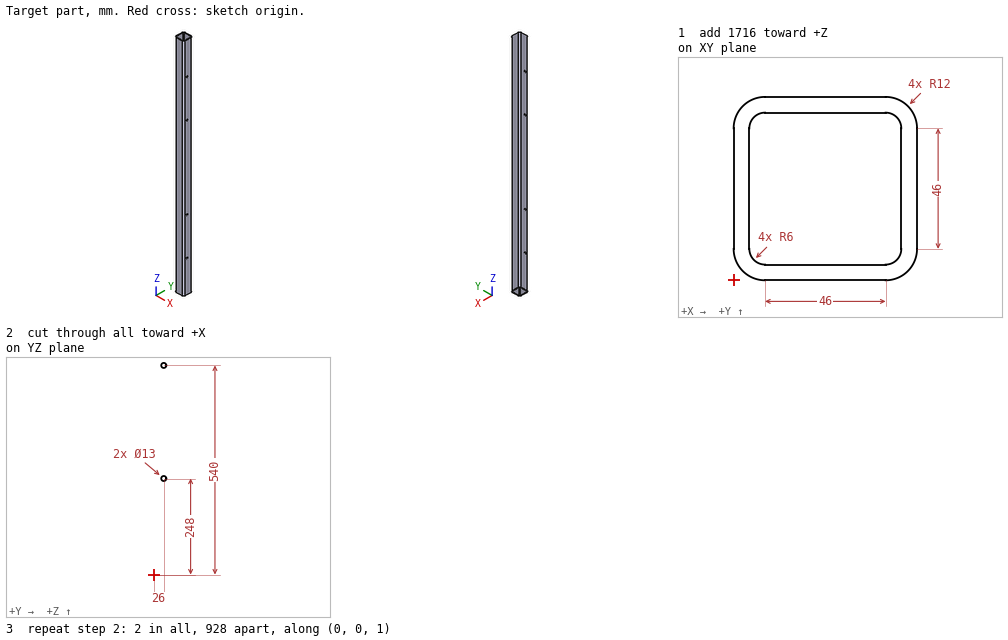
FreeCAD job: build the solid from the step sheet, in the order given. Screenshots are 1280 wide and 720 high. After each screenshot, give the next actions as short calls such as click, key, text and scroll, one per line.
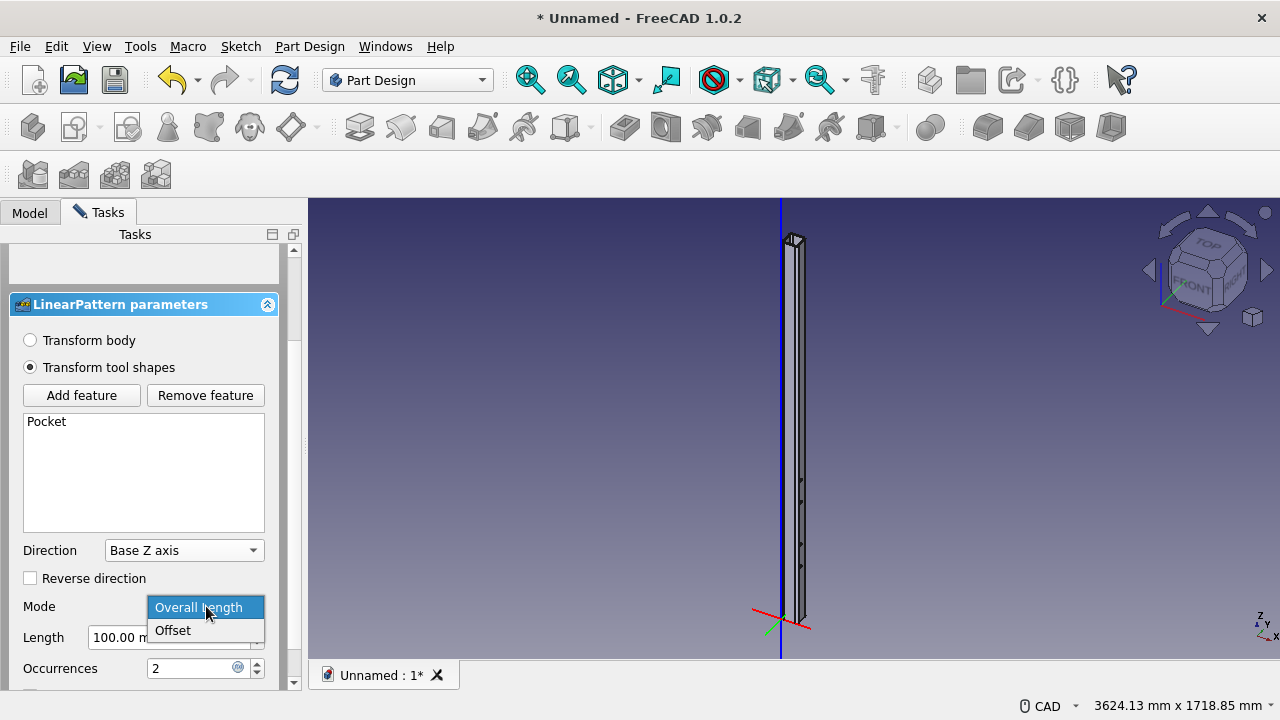
click(204, 630)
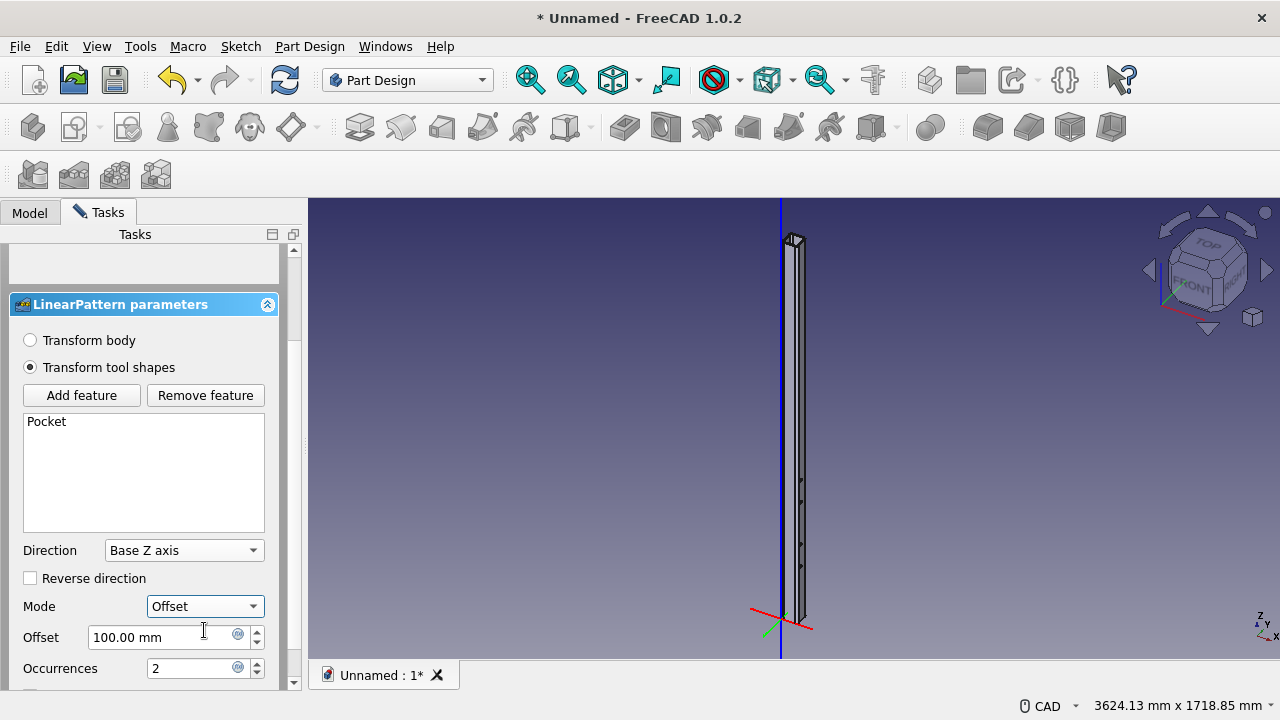
triple_click(170, 638)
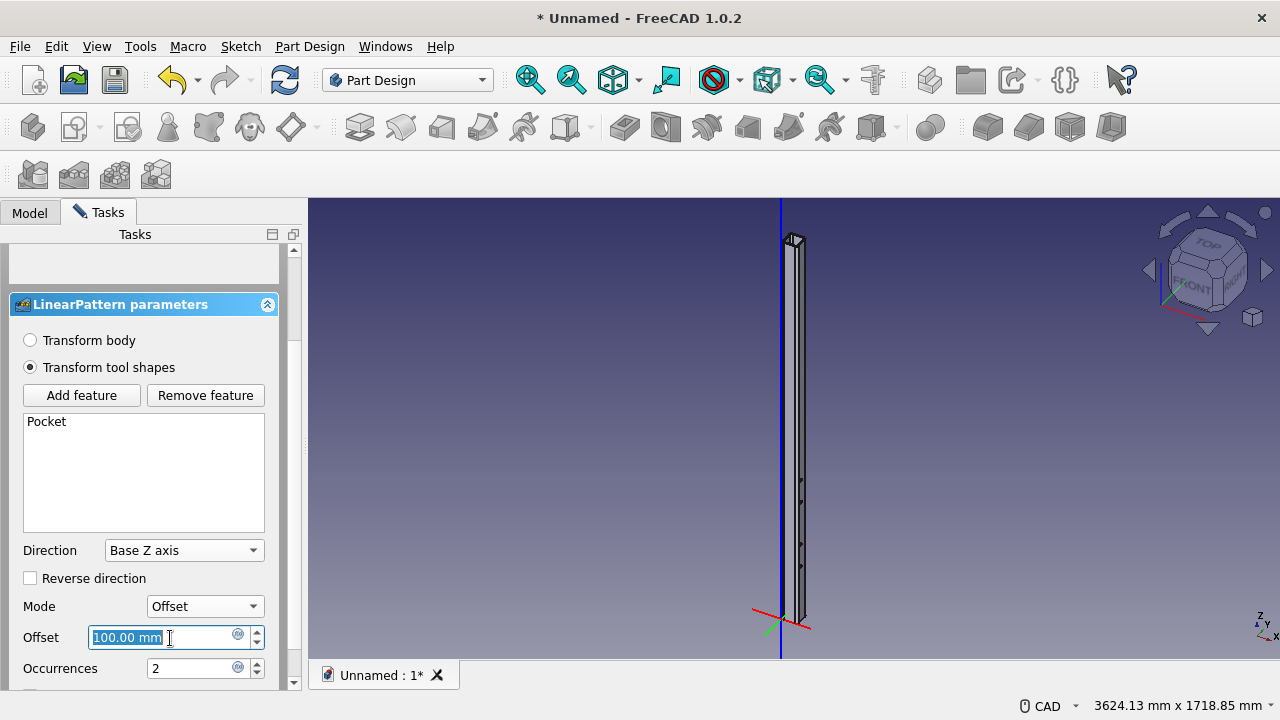
text(928)
key(Tab)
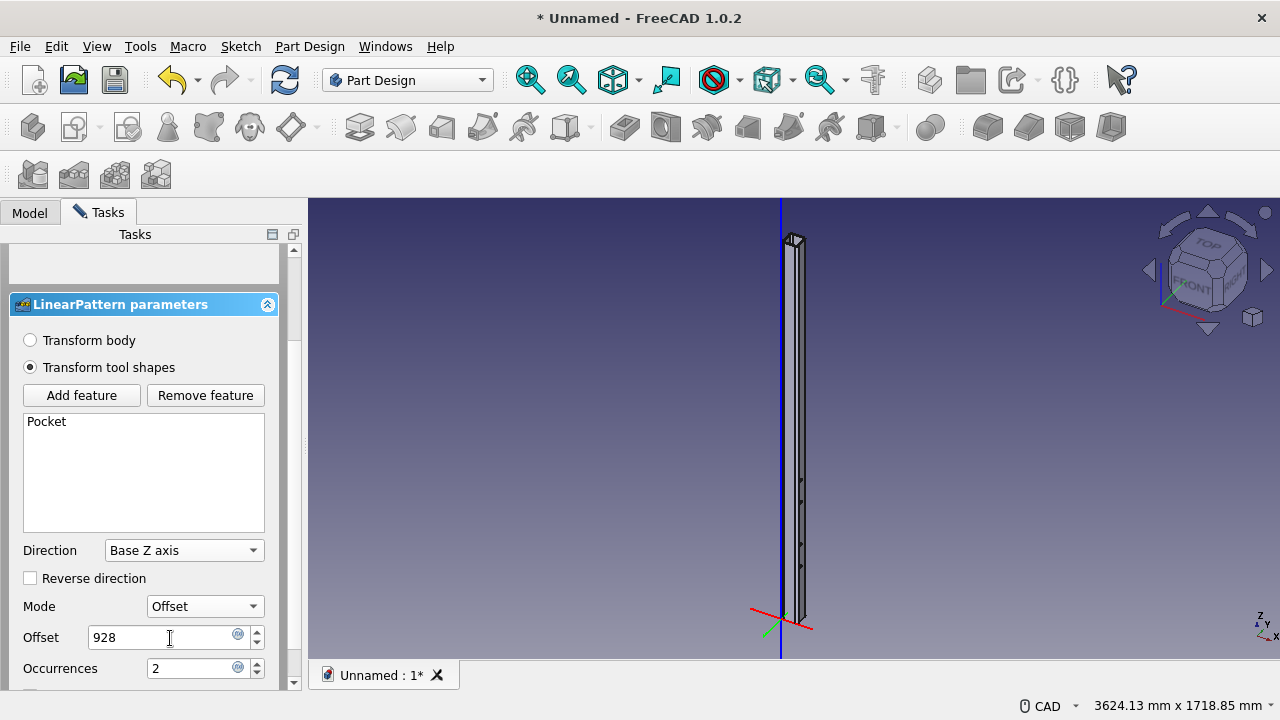
triple_click(199, 668)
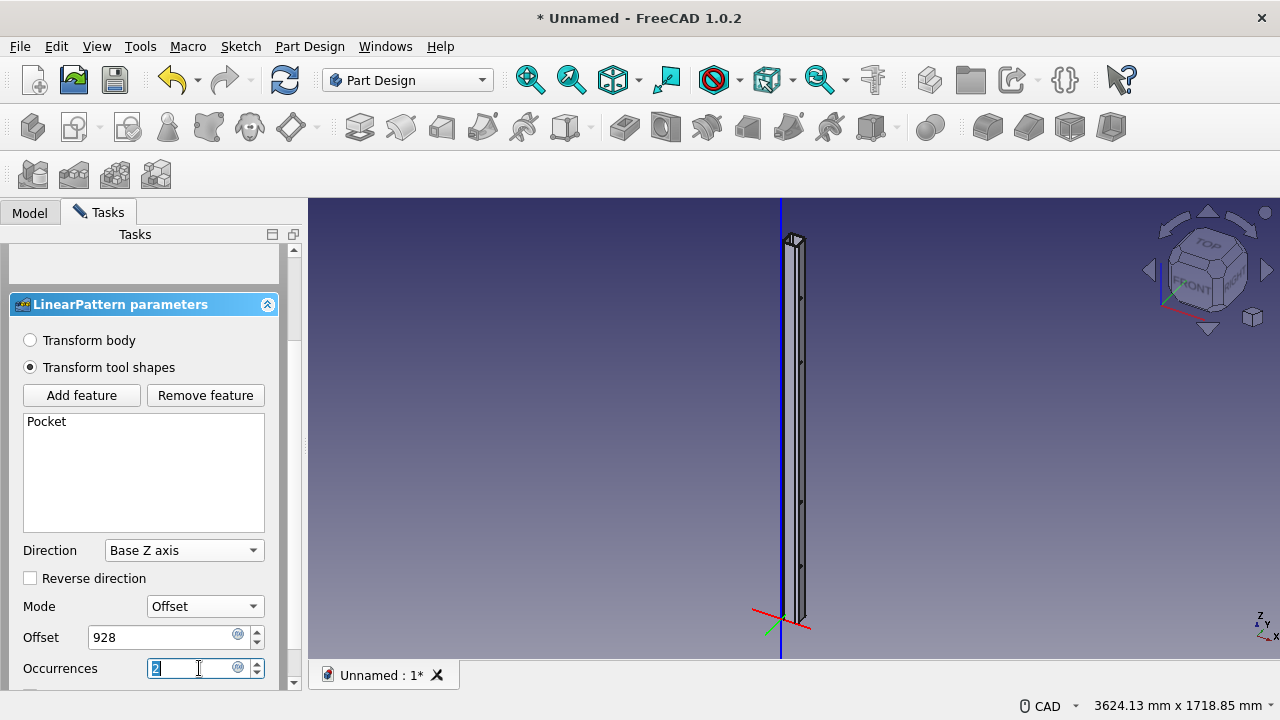
text(2)
key(Tab)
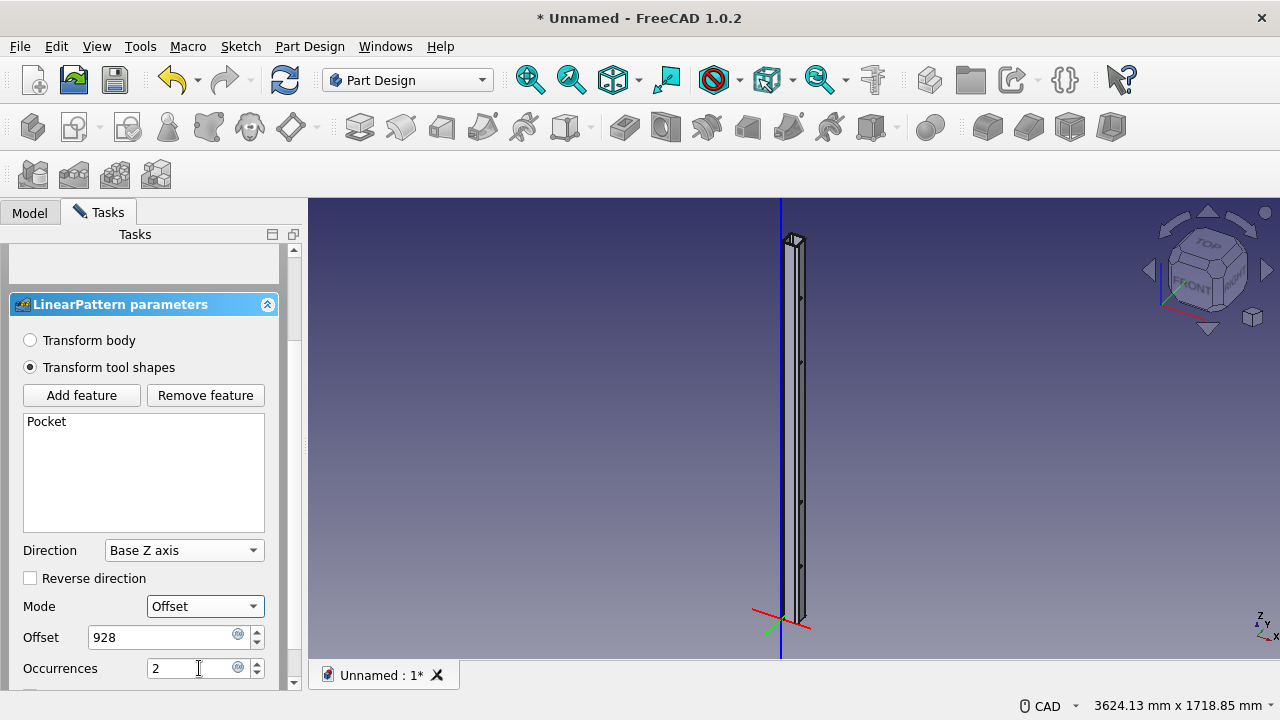
scroll(294, 467, up, 3)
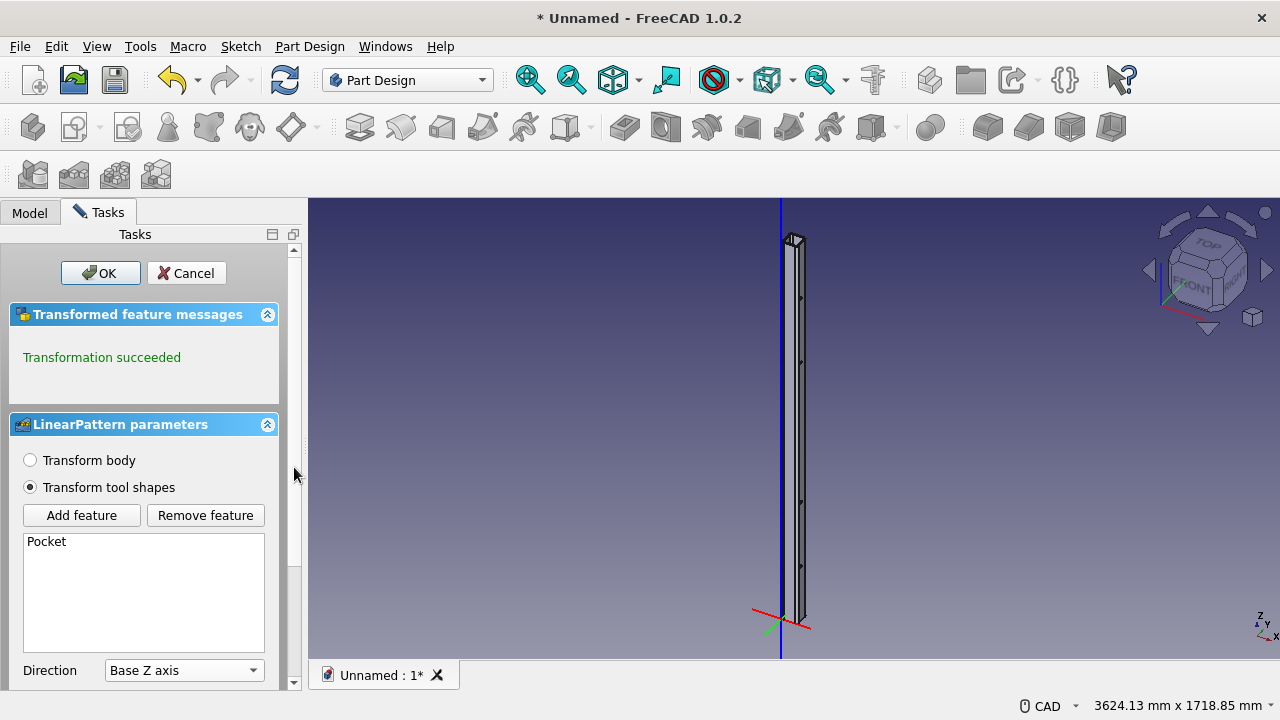
click(101, 273)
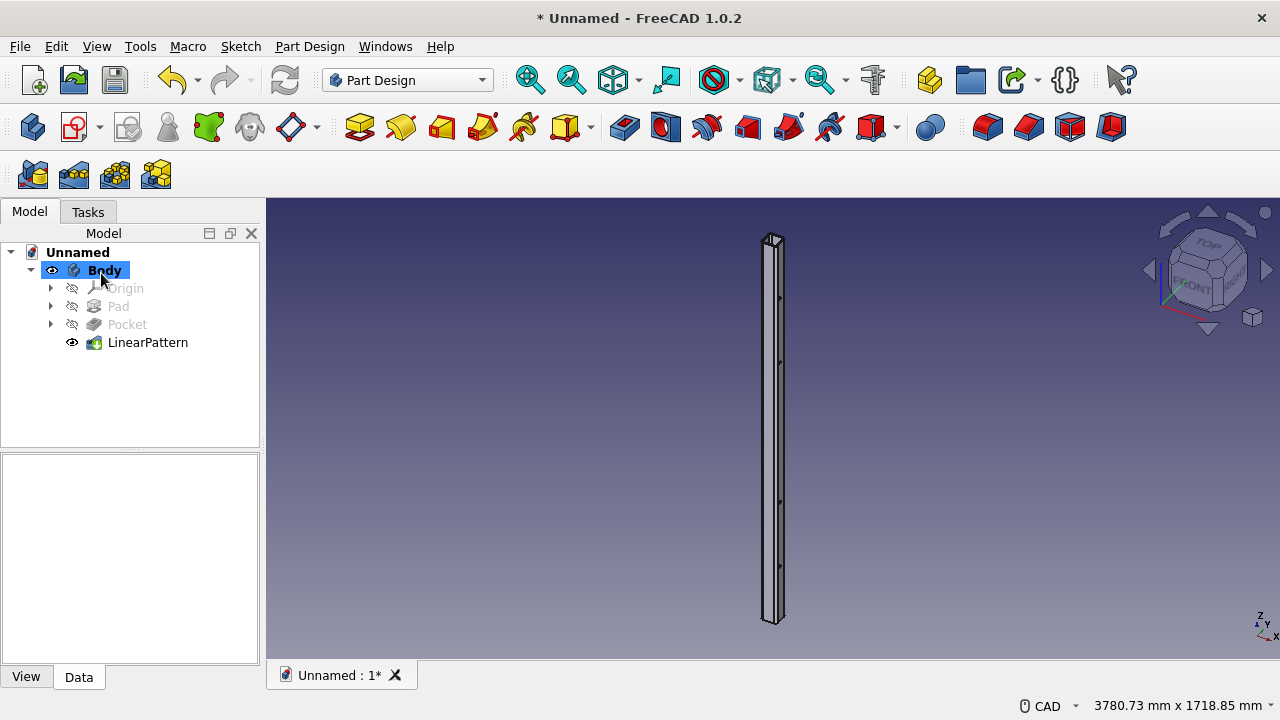
key(0)